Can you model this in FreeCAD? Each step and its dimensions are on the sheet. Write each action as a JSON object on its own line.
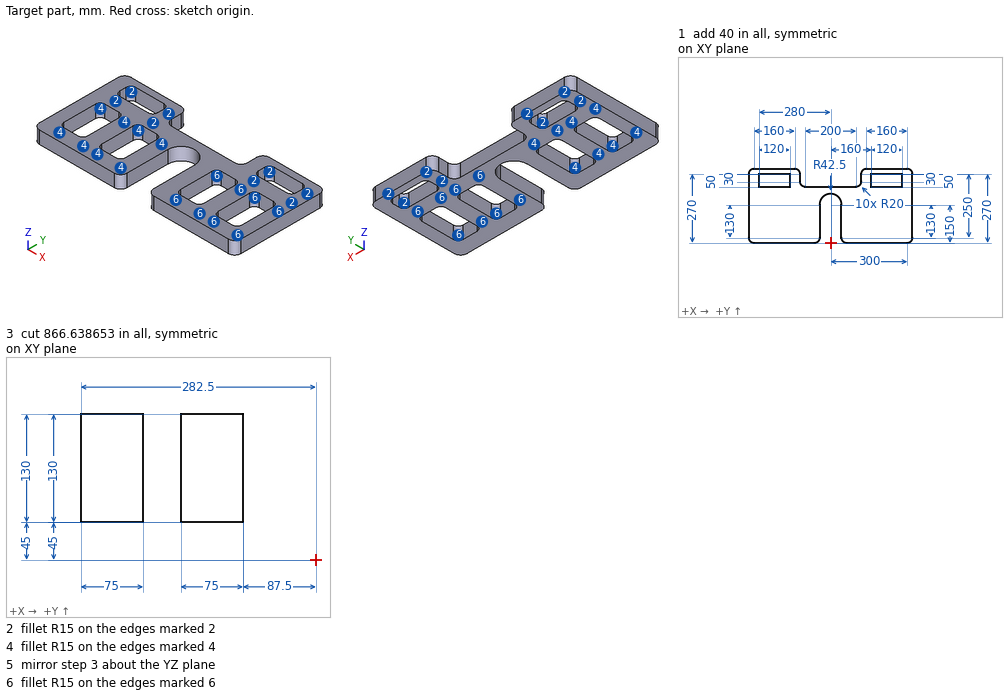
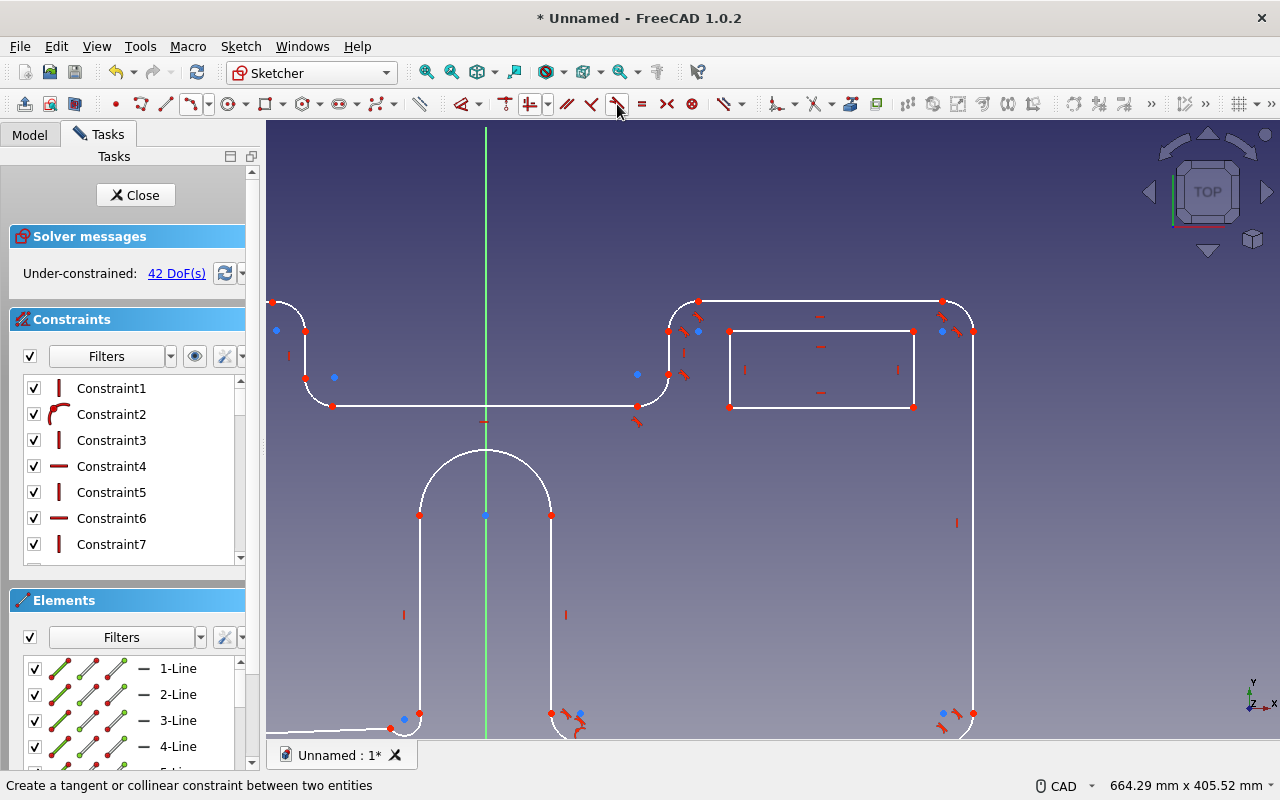
{"action": "left_click", "coordinate": [546, 406]}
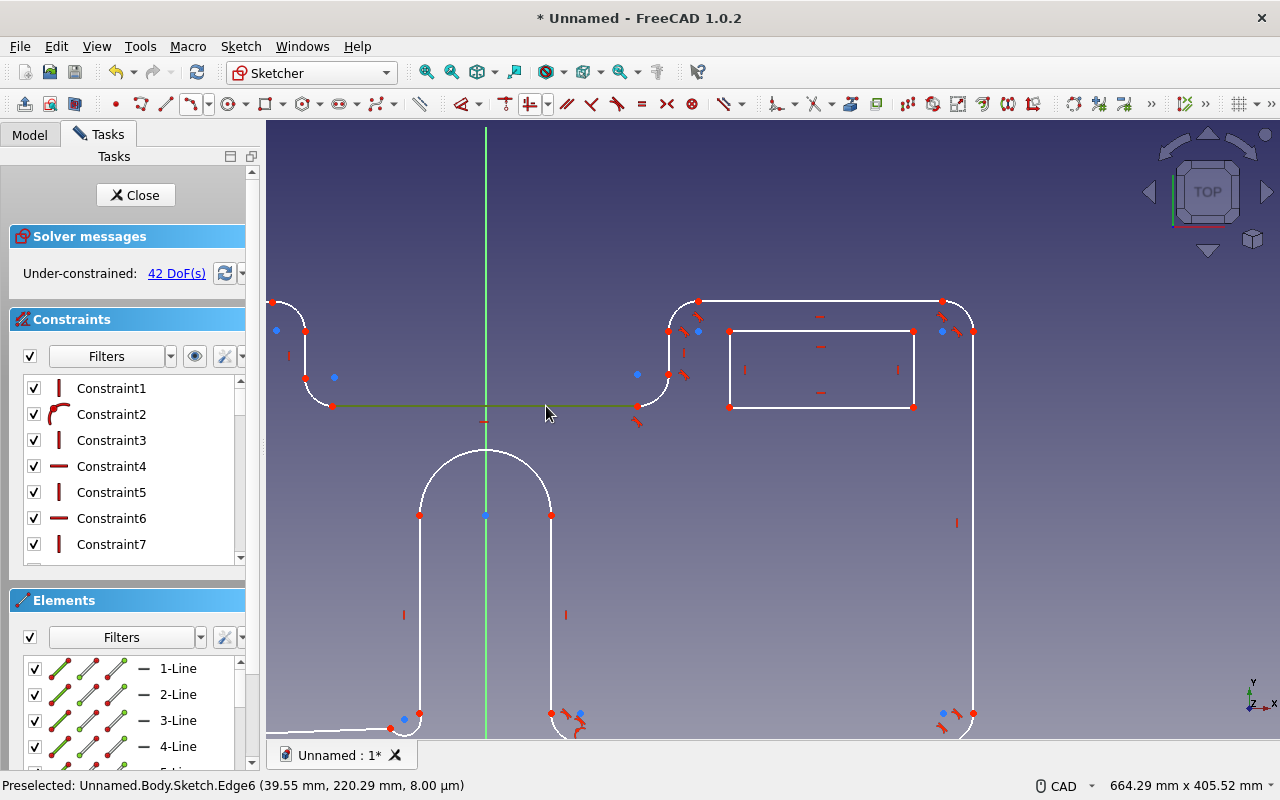
{"action": "left_click", "coordinate": [308, 391]}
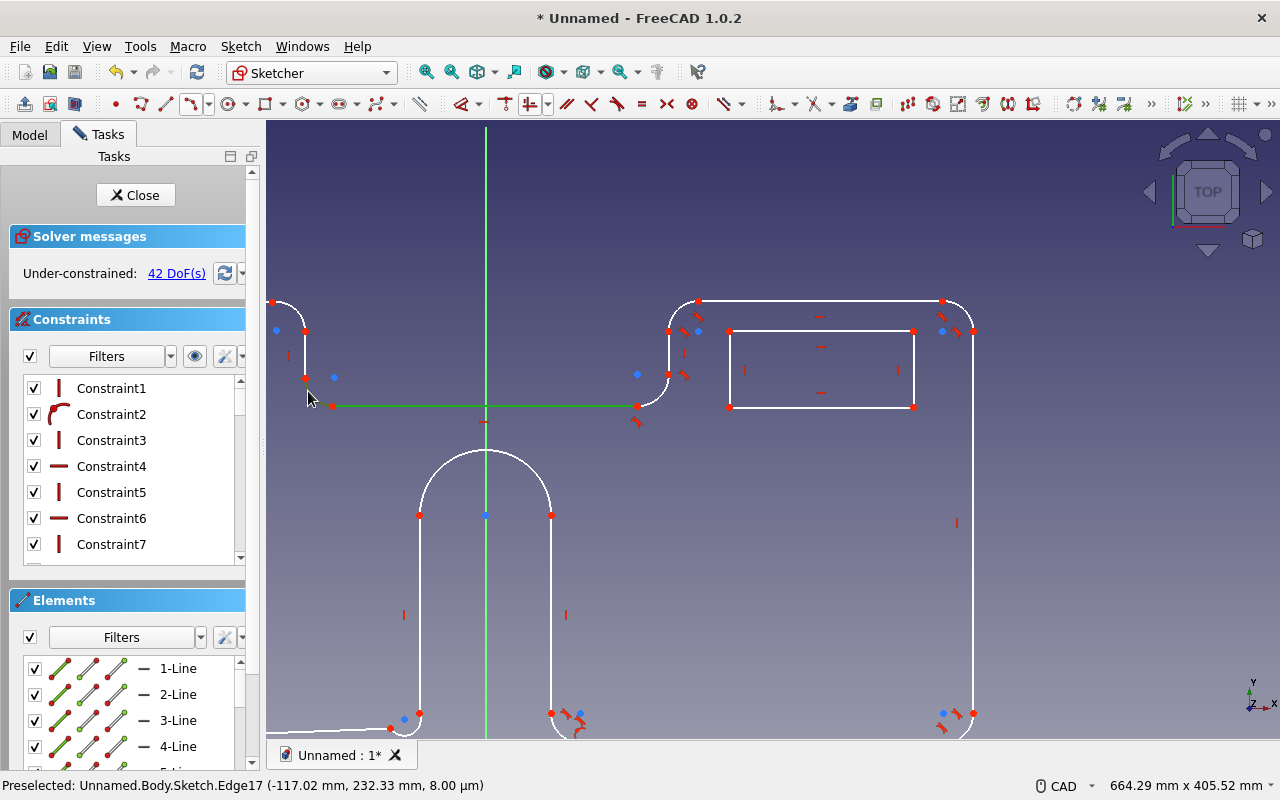
{"action": "left_click", "coordinate": [617, 104]}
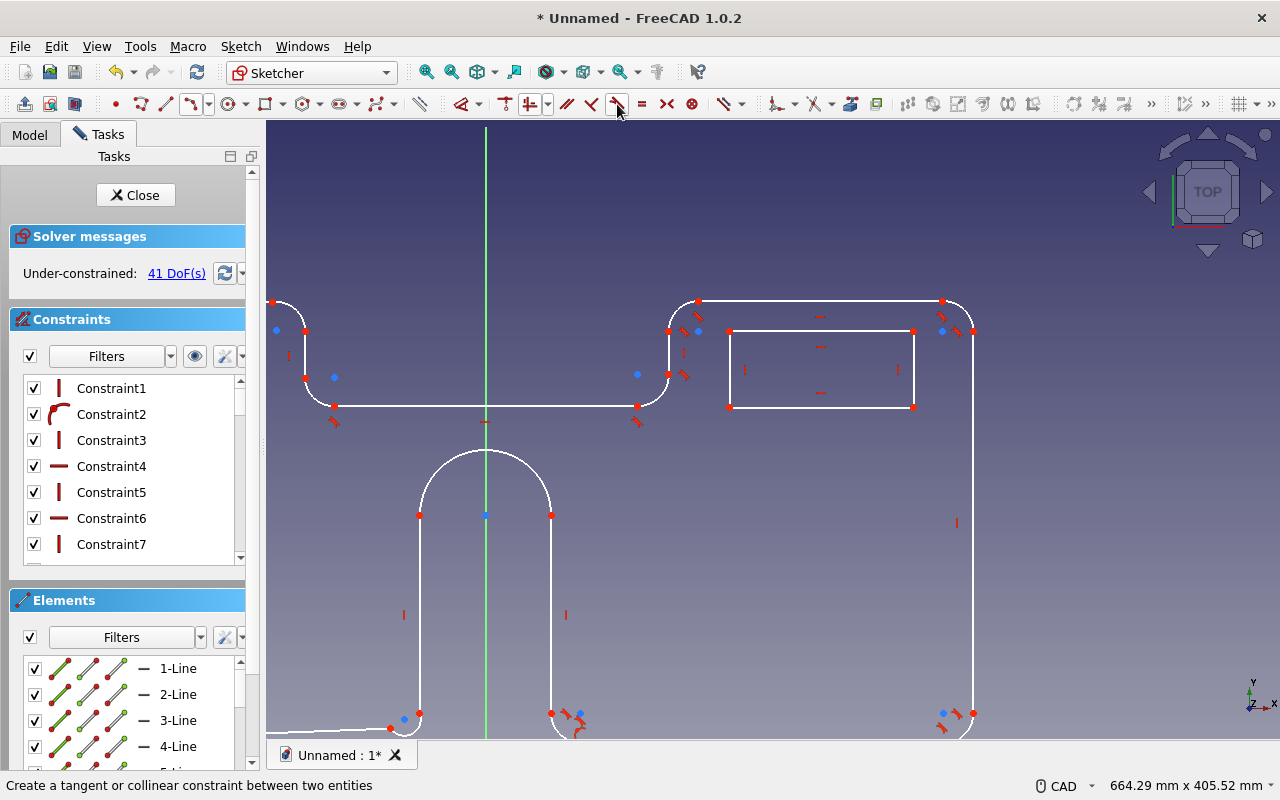
{"action": "left_click", "coordinate": [305, 364]}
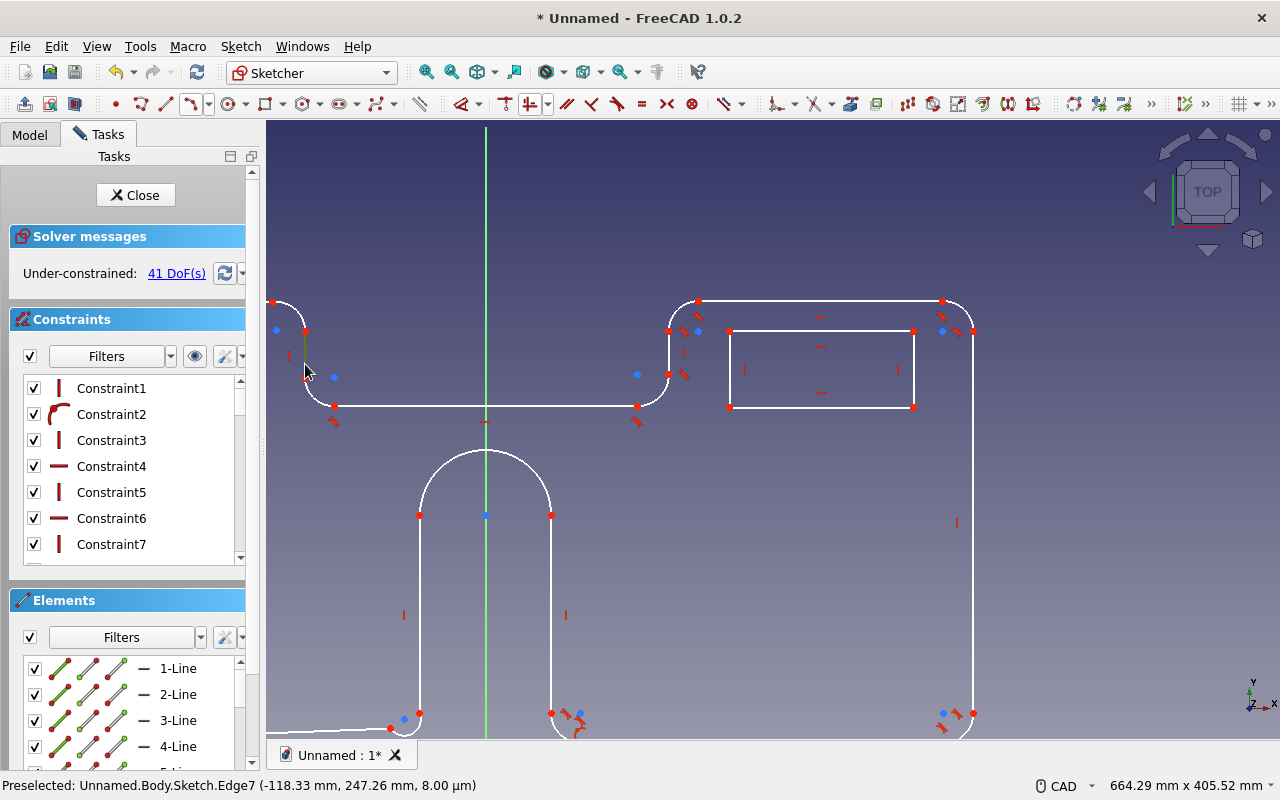
{"action": "left_click", "coordinate": [309, 391]}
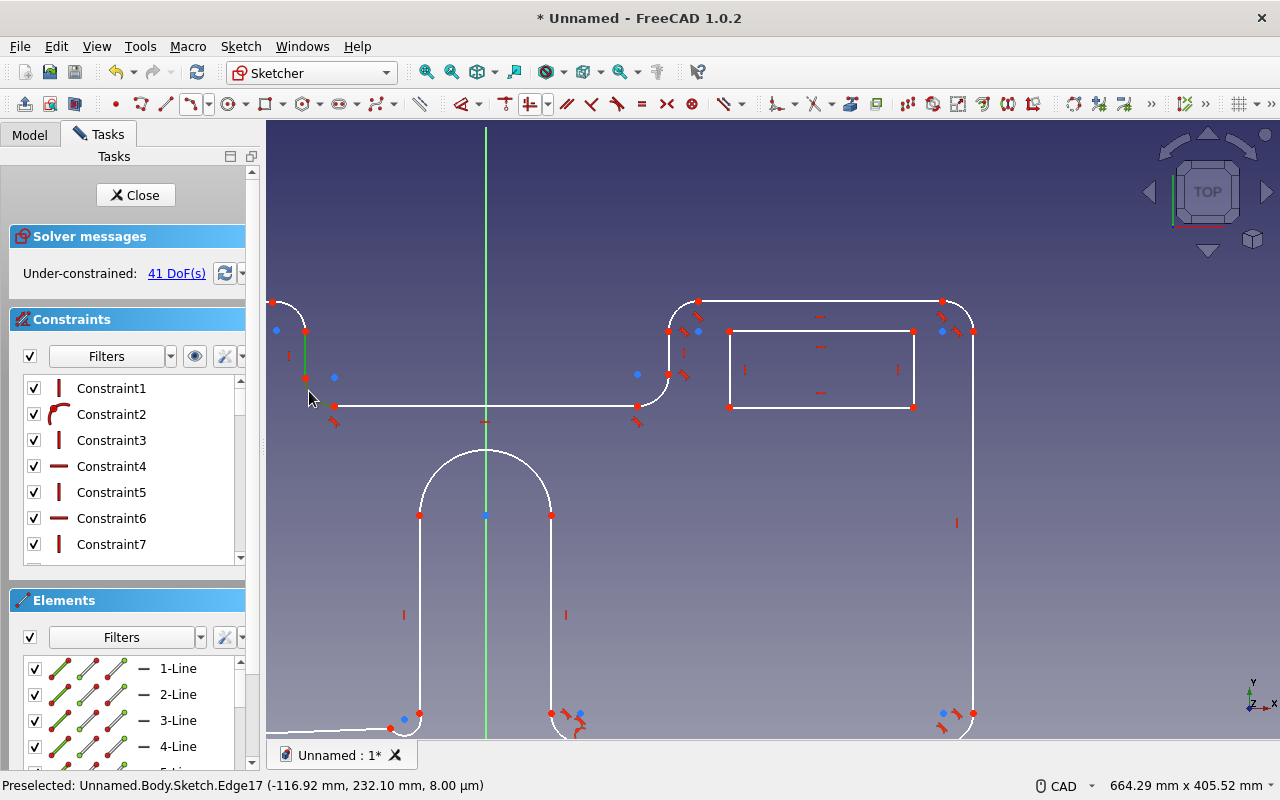
{"action": "key", "text": "t"}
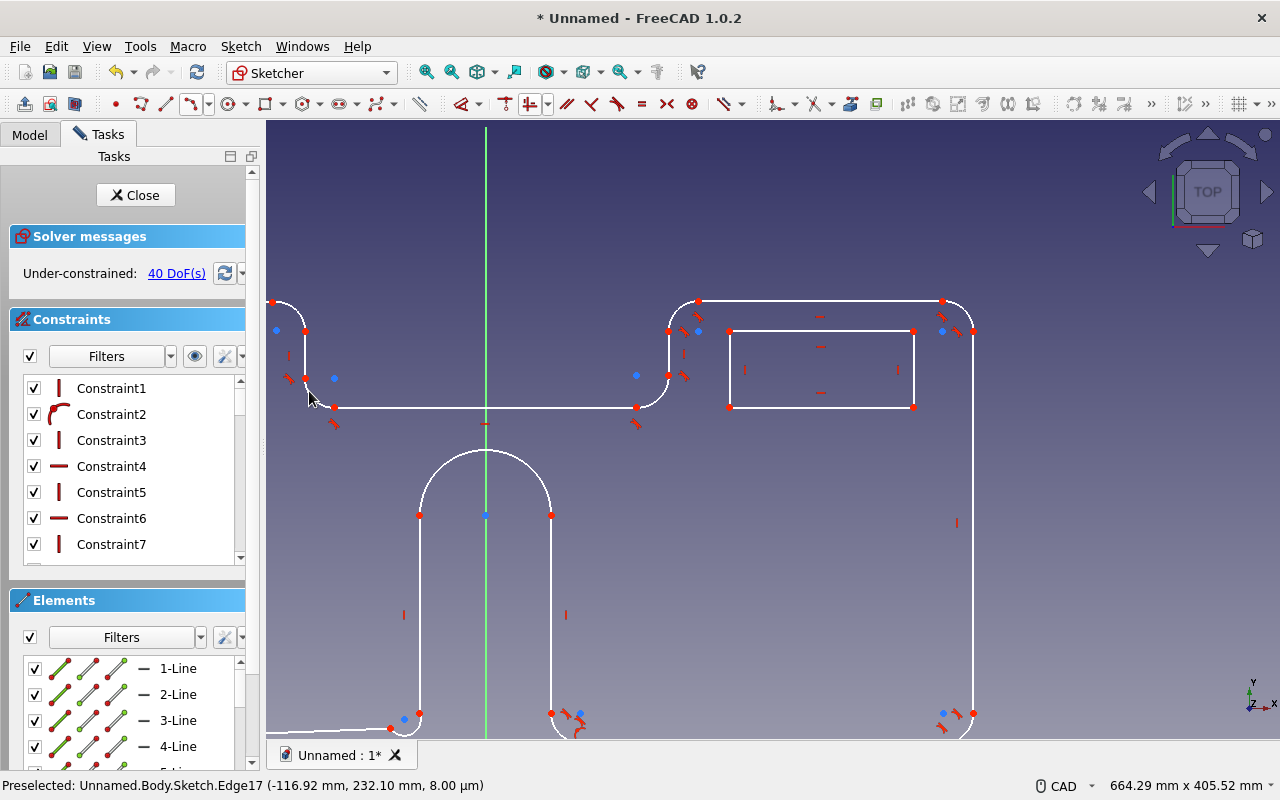
{"action": "left_click", "coordinate": [305, 364]}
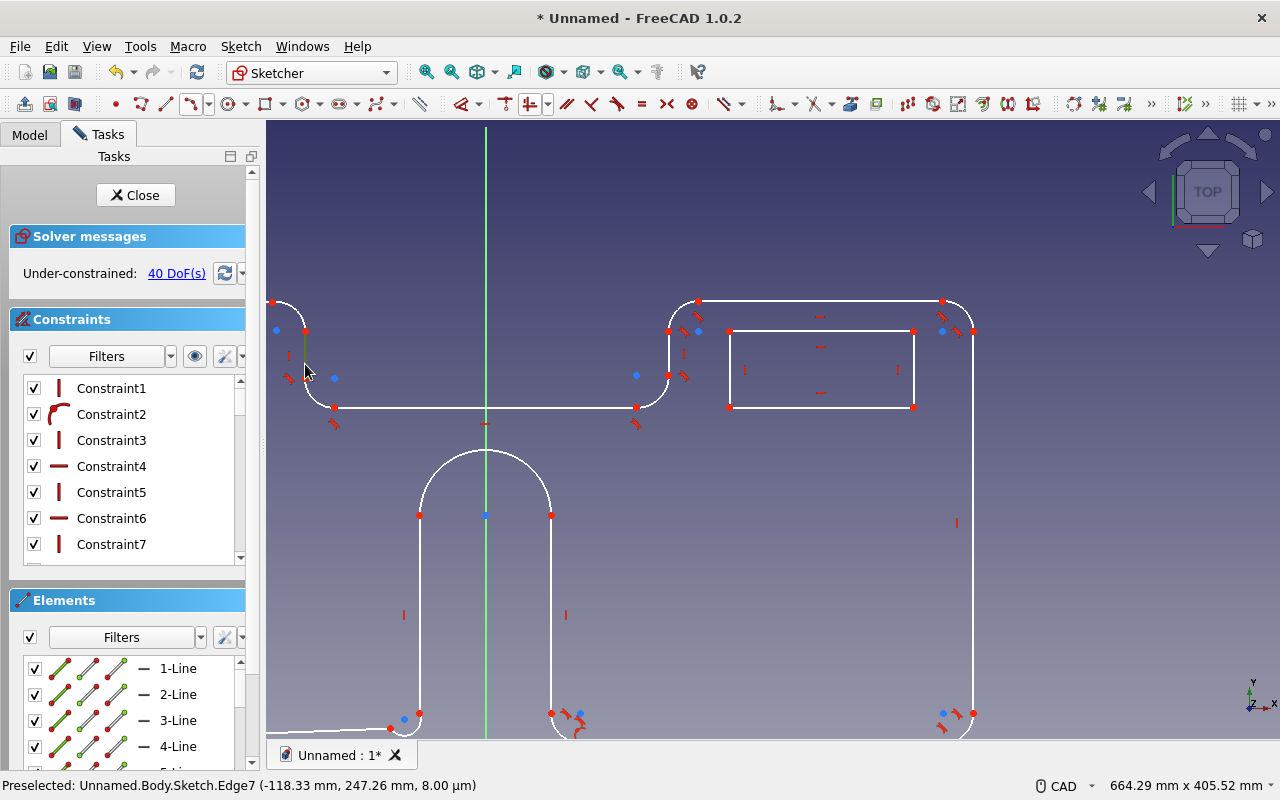
{"action": "left_click", "coordinate": [301, 317]}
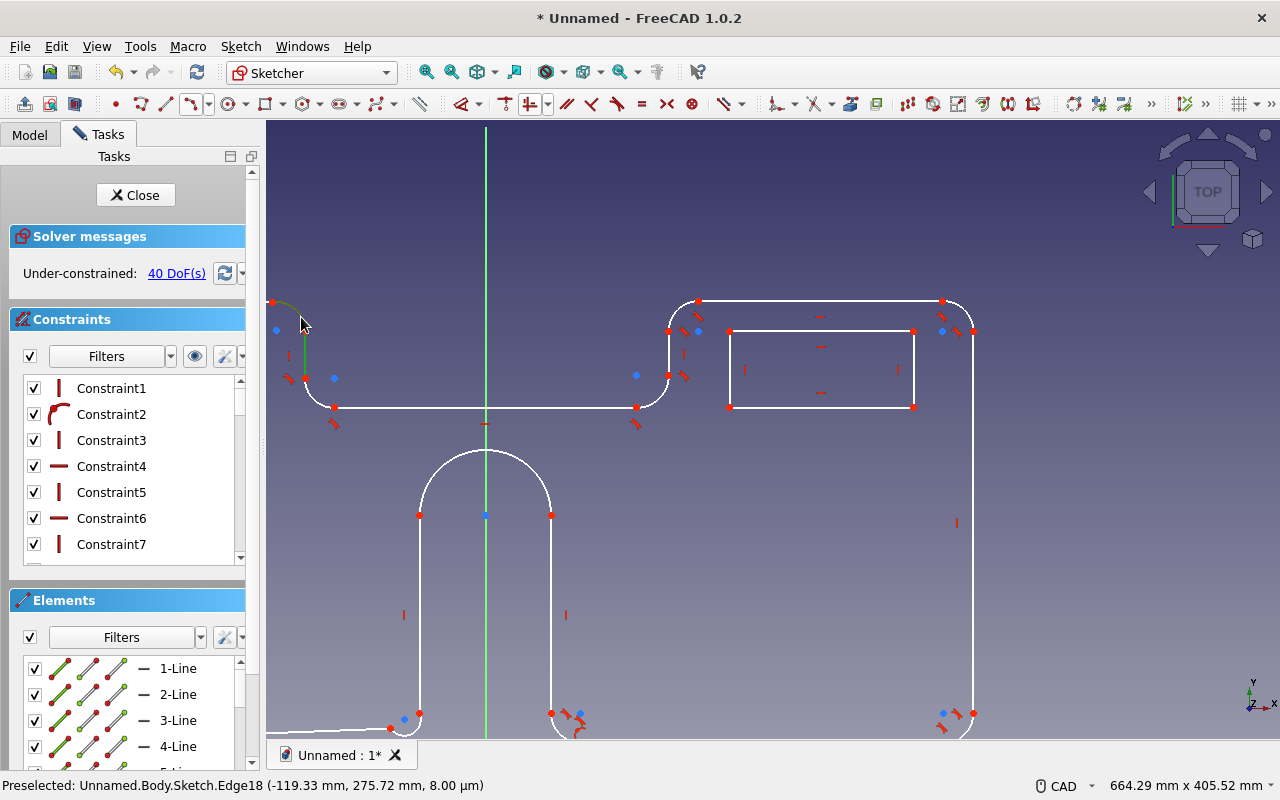
{"action": "key", "text": "t"}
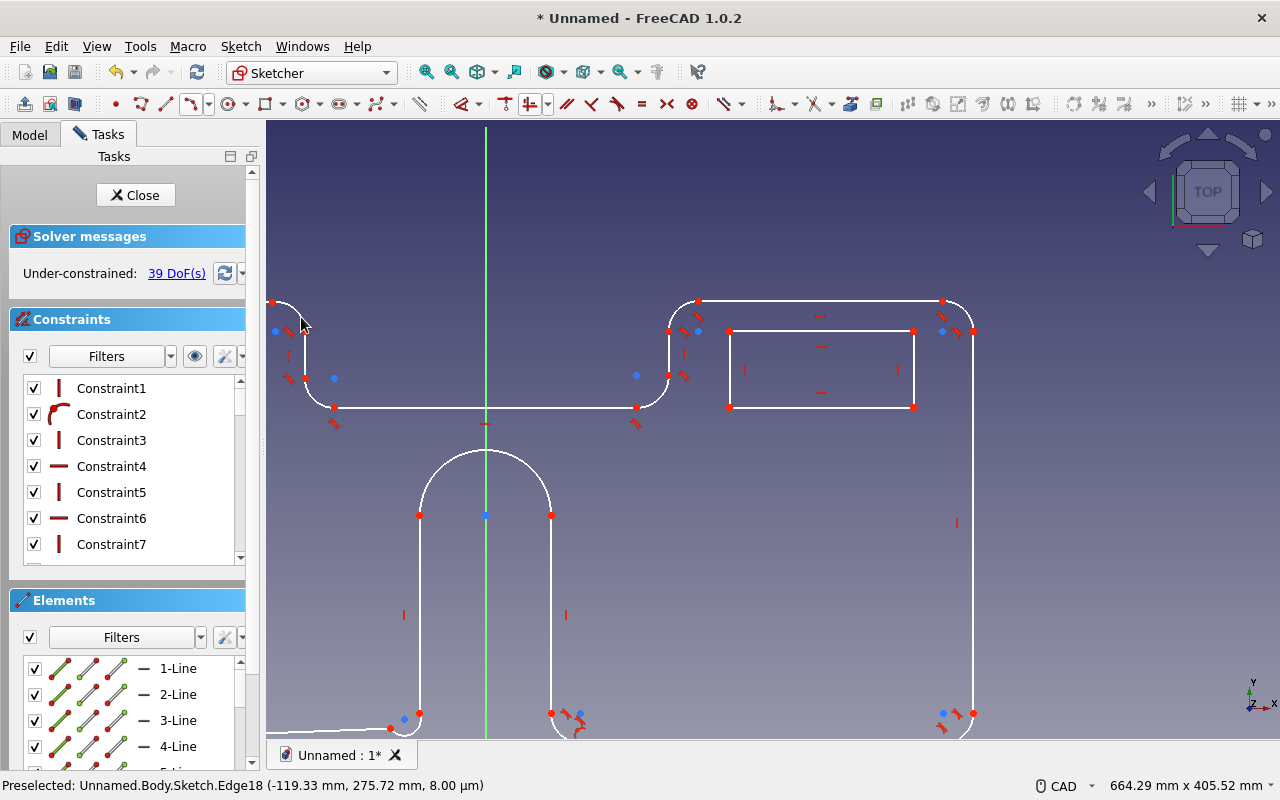
{"action": "scroll", "coordinate": [971, 318], "scroll_direction": "down", "scroll_amount": 3}